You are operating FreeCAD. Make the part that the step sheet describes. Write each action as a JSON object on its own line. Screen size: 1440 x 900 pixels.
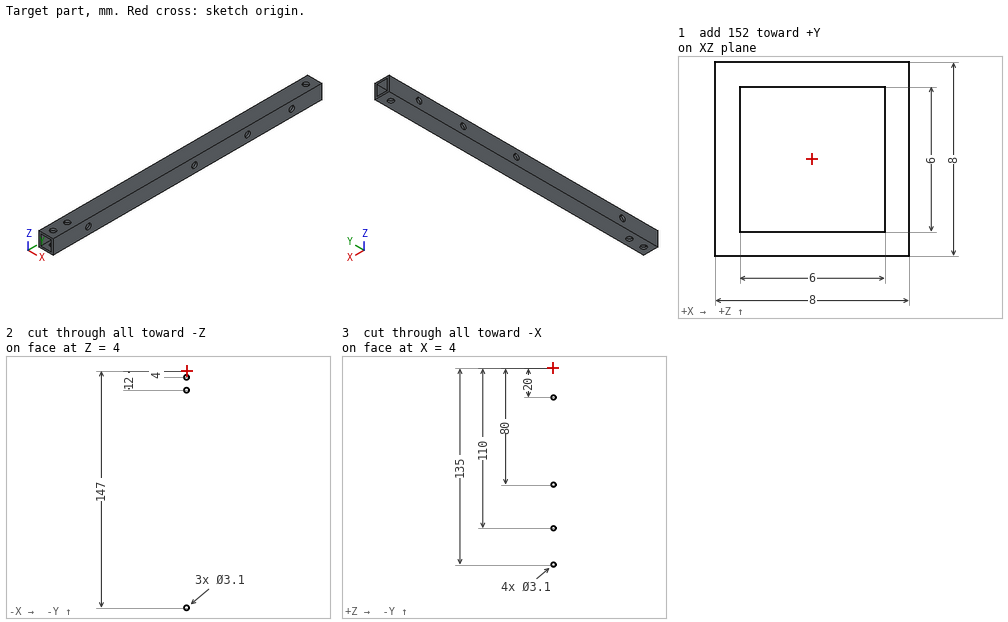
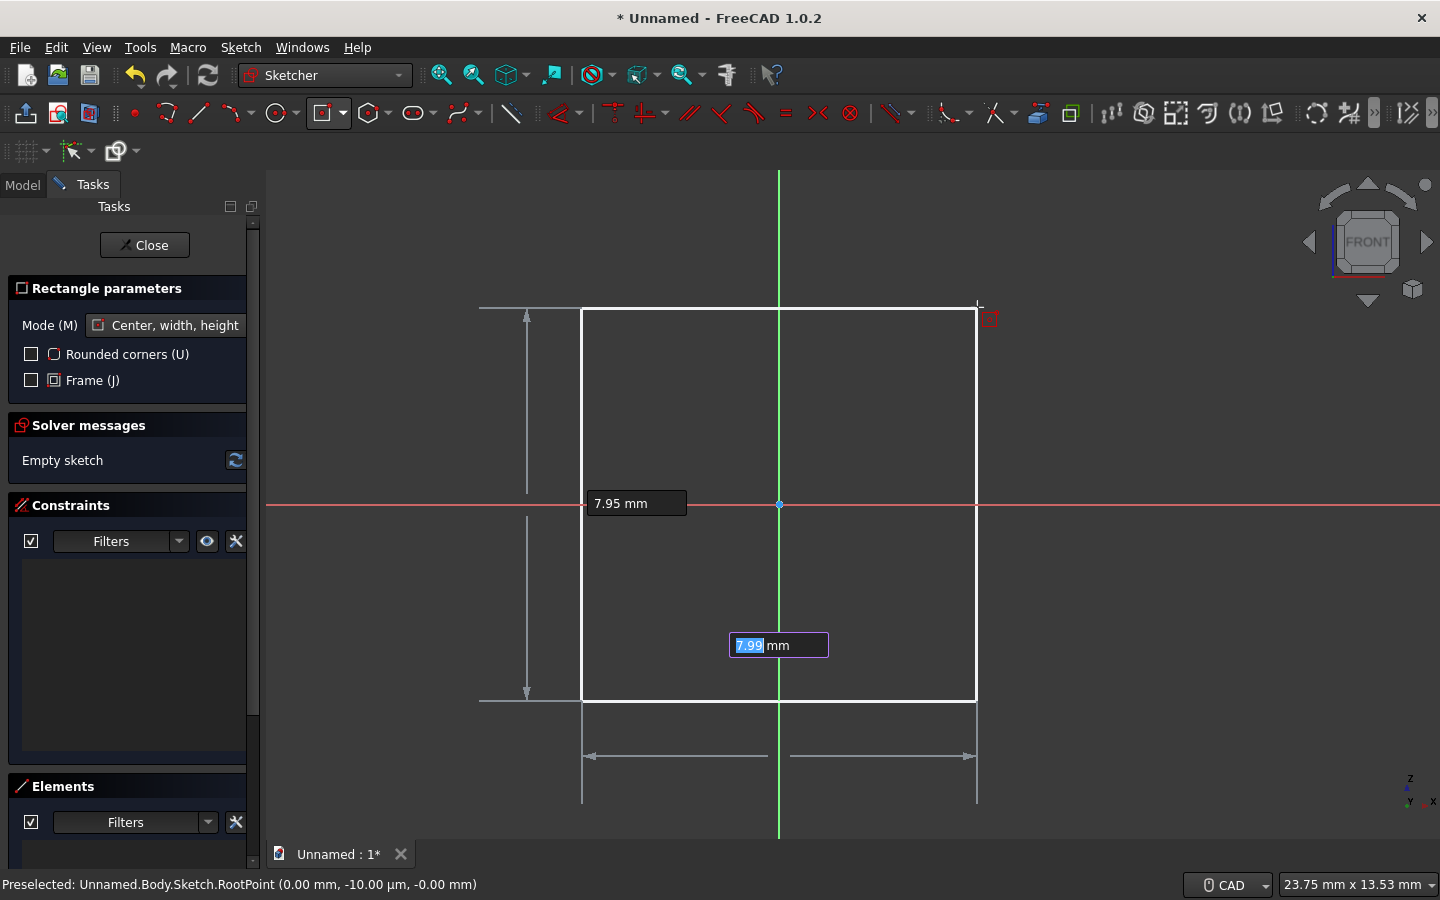
{"action": "type", "text": "8"}
{"action": "key", "text": "Tab"}
{"action": "type", "text": "8"}
{"action": "key", "text": "Return"}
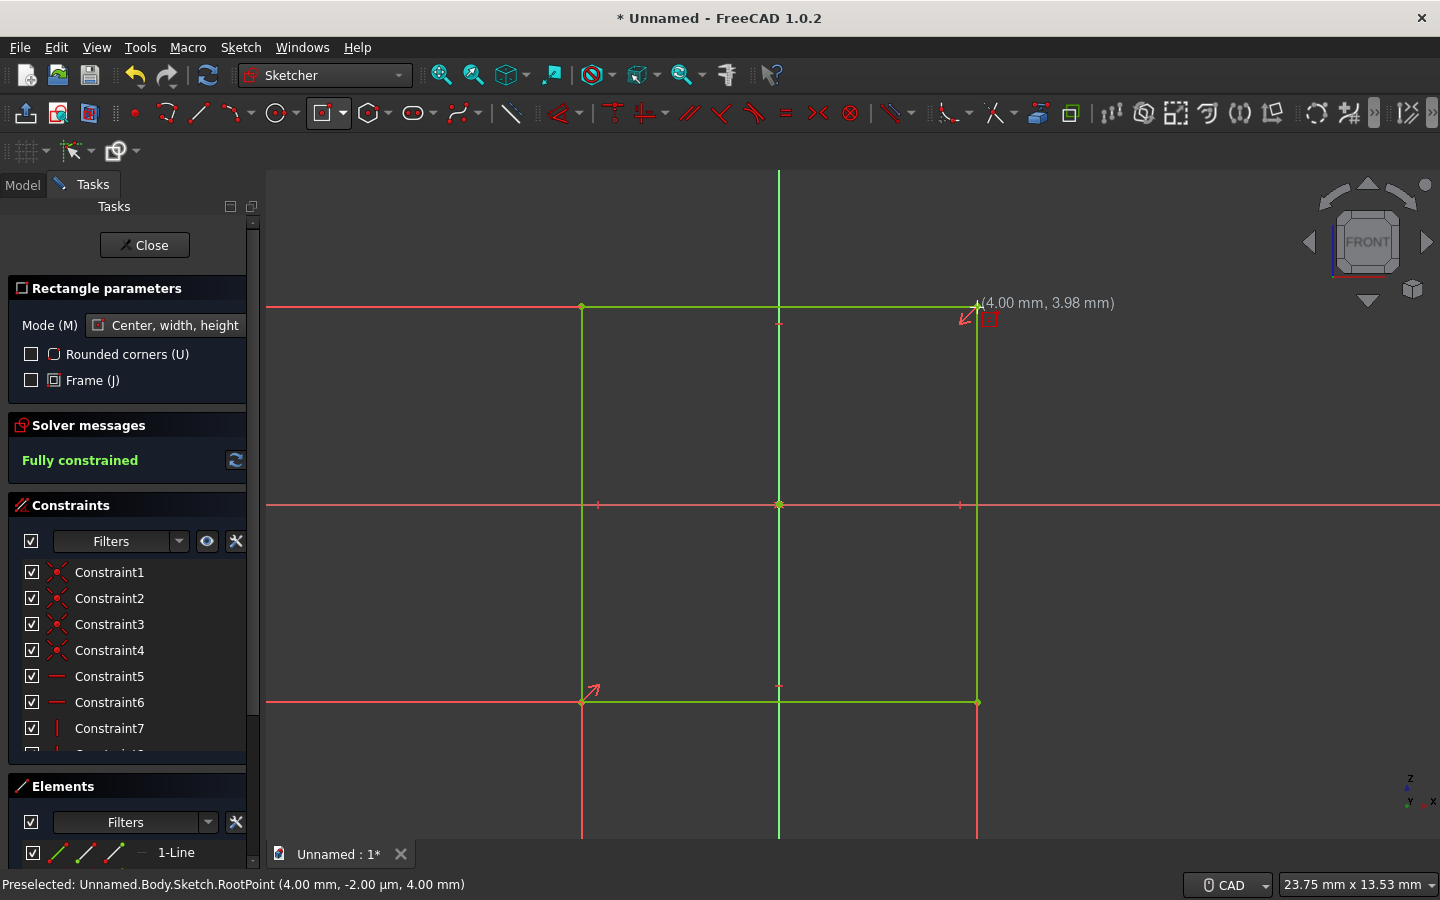
{"action": "left_click", "coordinate": [779, 504]}
{"action": "mouse_move", "coordinate": [928, 356]}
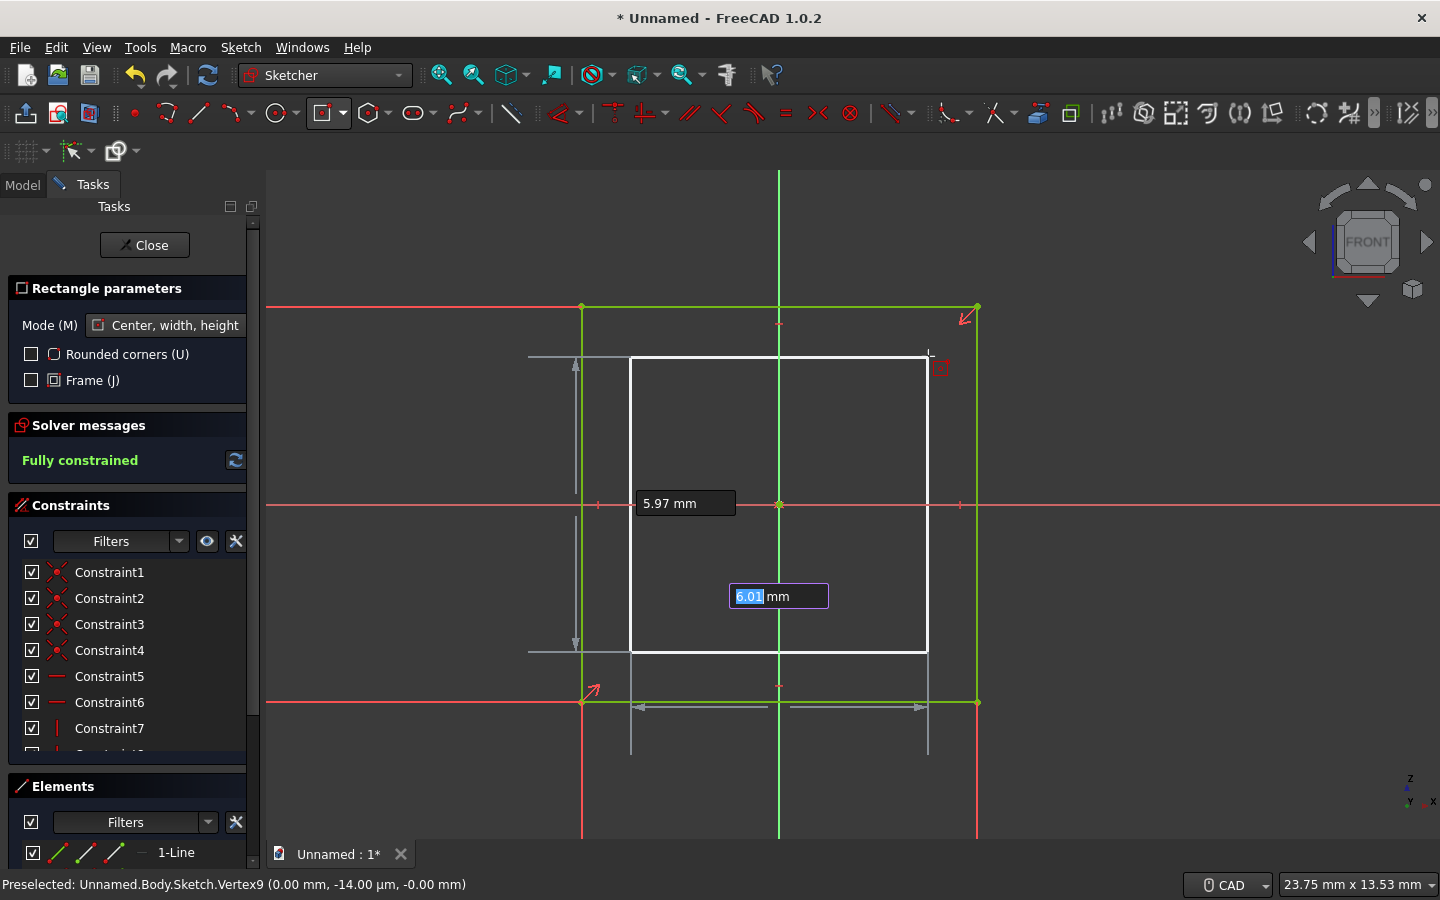
{"action": "type", "text": "6"}
{"action": "key", "text": "Tab"}
{"action": "type", "text": "6"}
{"action": "key", "text": "Return"}
{"action": "key", "text": "Escape"}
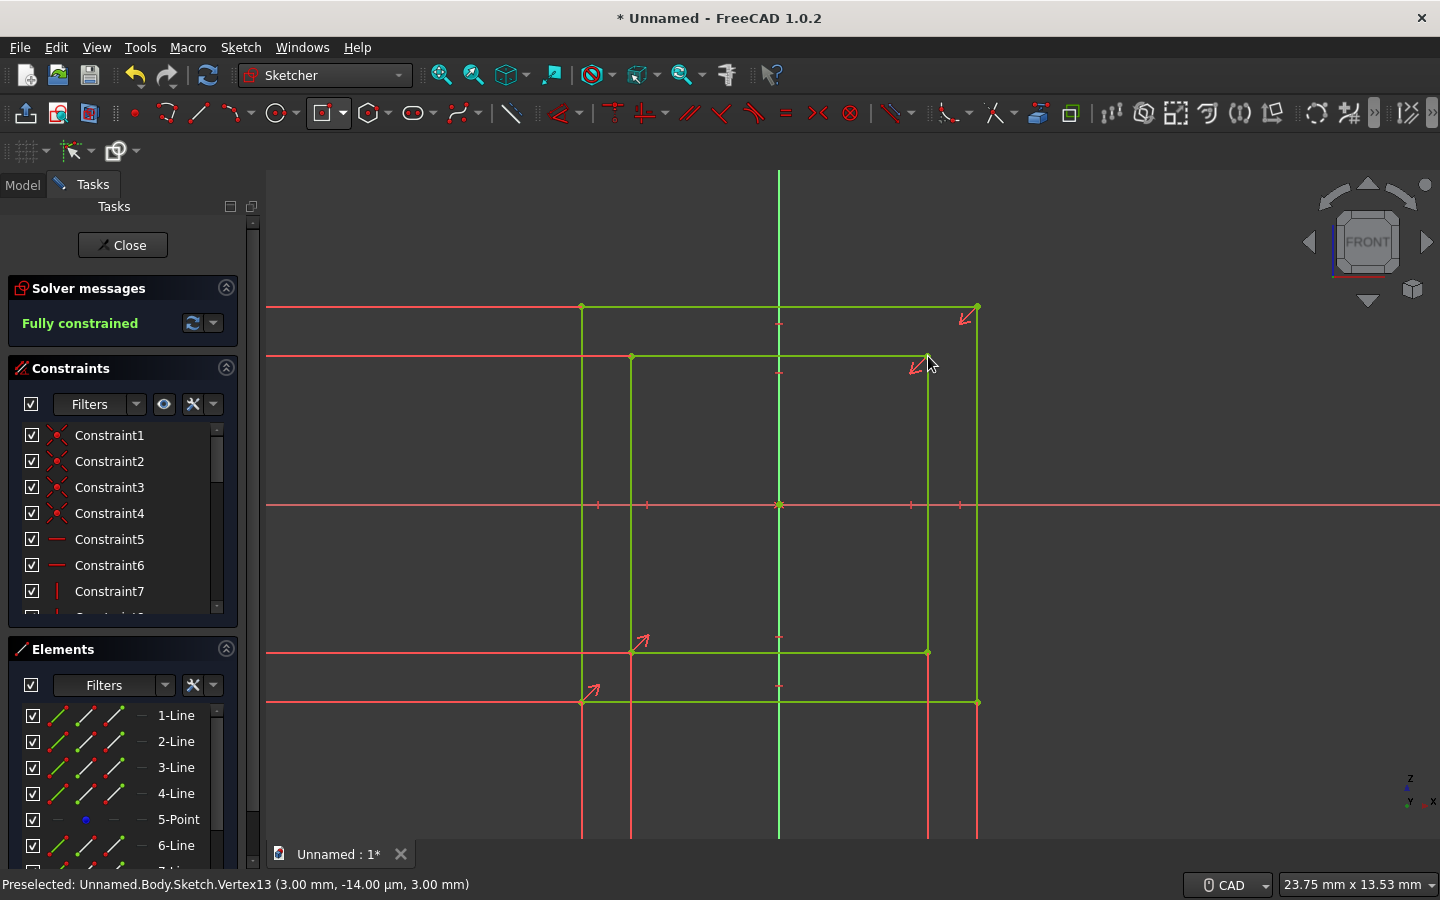
{"action": "left_click", "coordinate": [123, 245]}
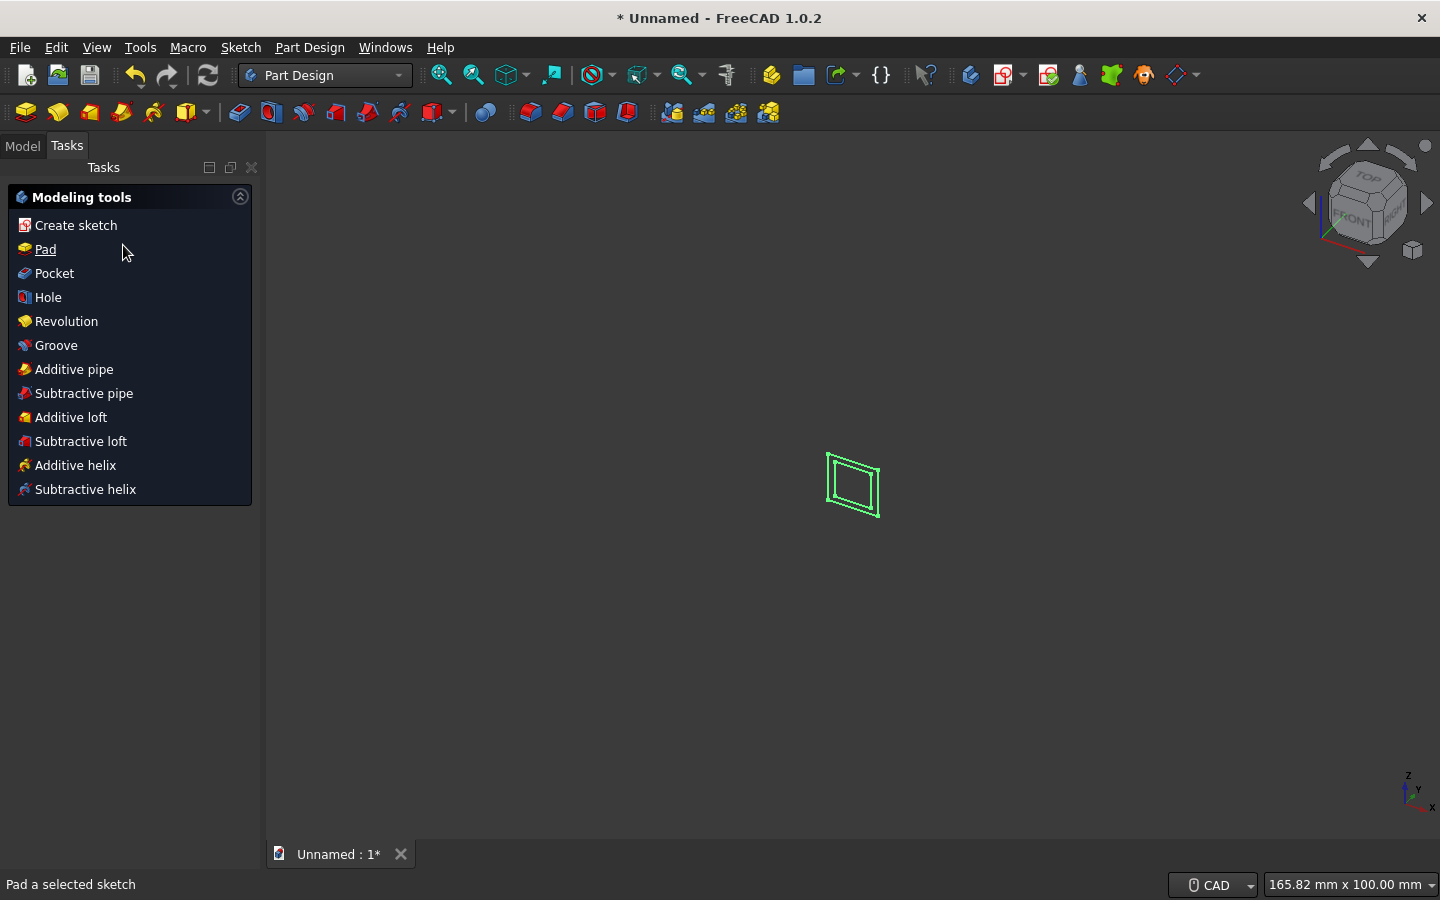
{"action": "left_click", "coordinate": [26, 112]}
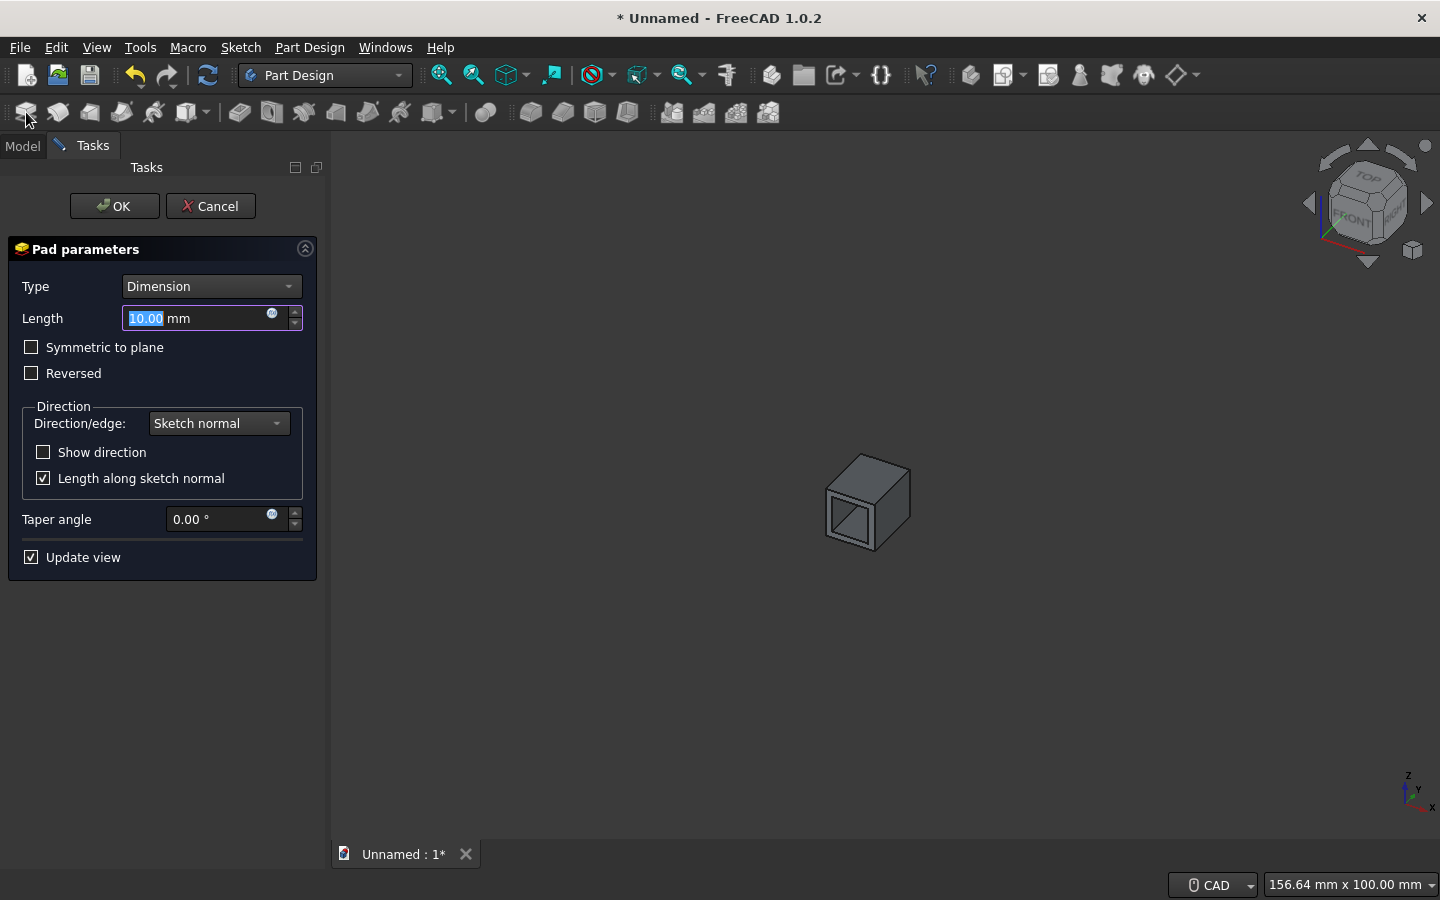
{"action": "type", "text": "152"}
{"action": "key", "text": "Tab"}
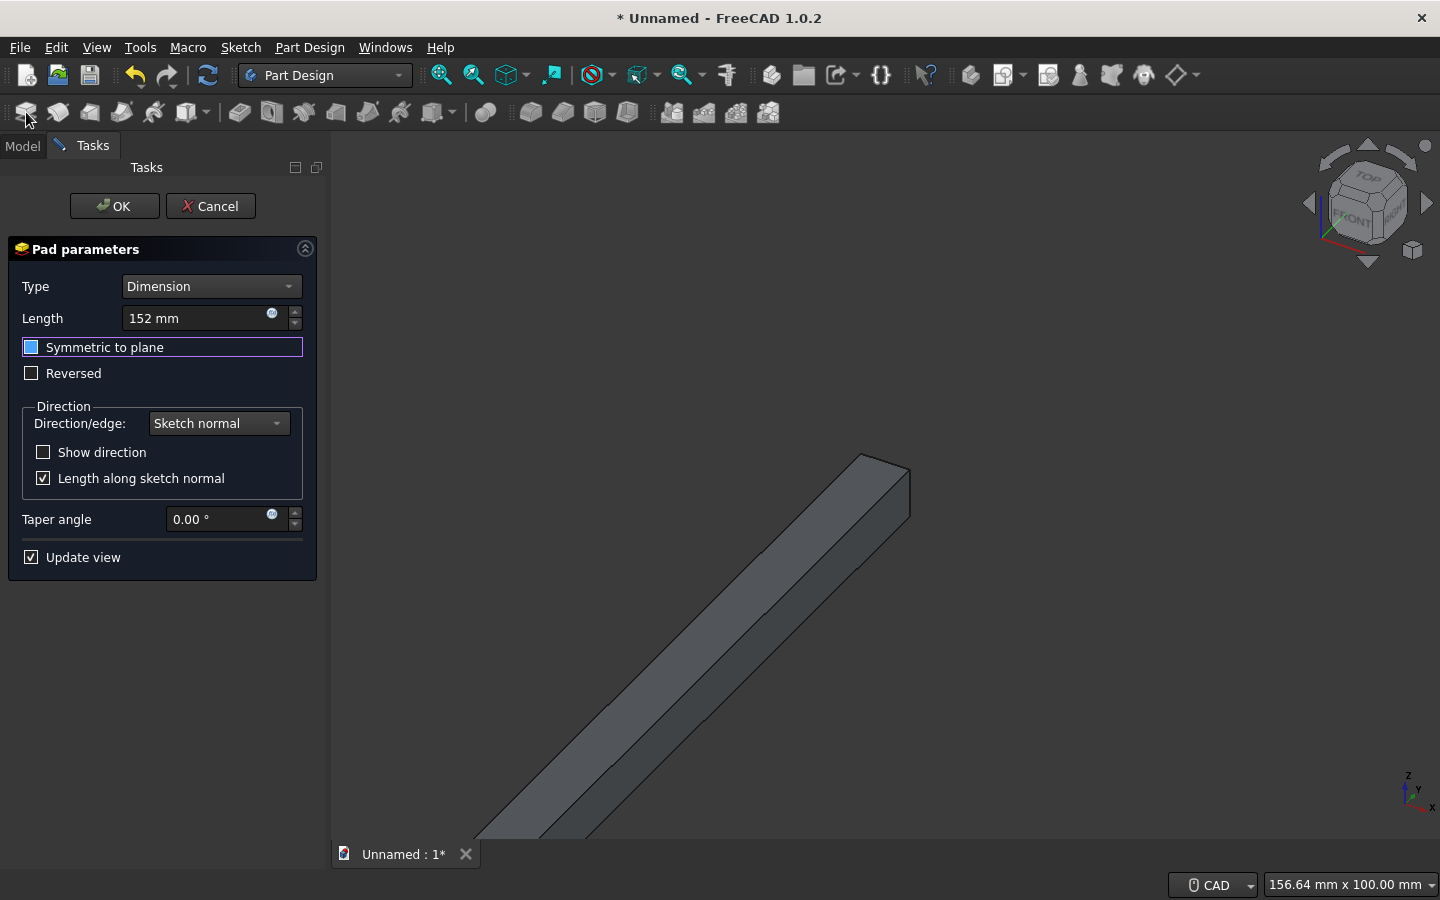
{"action": "left_click", "coordinate": [30, 373]}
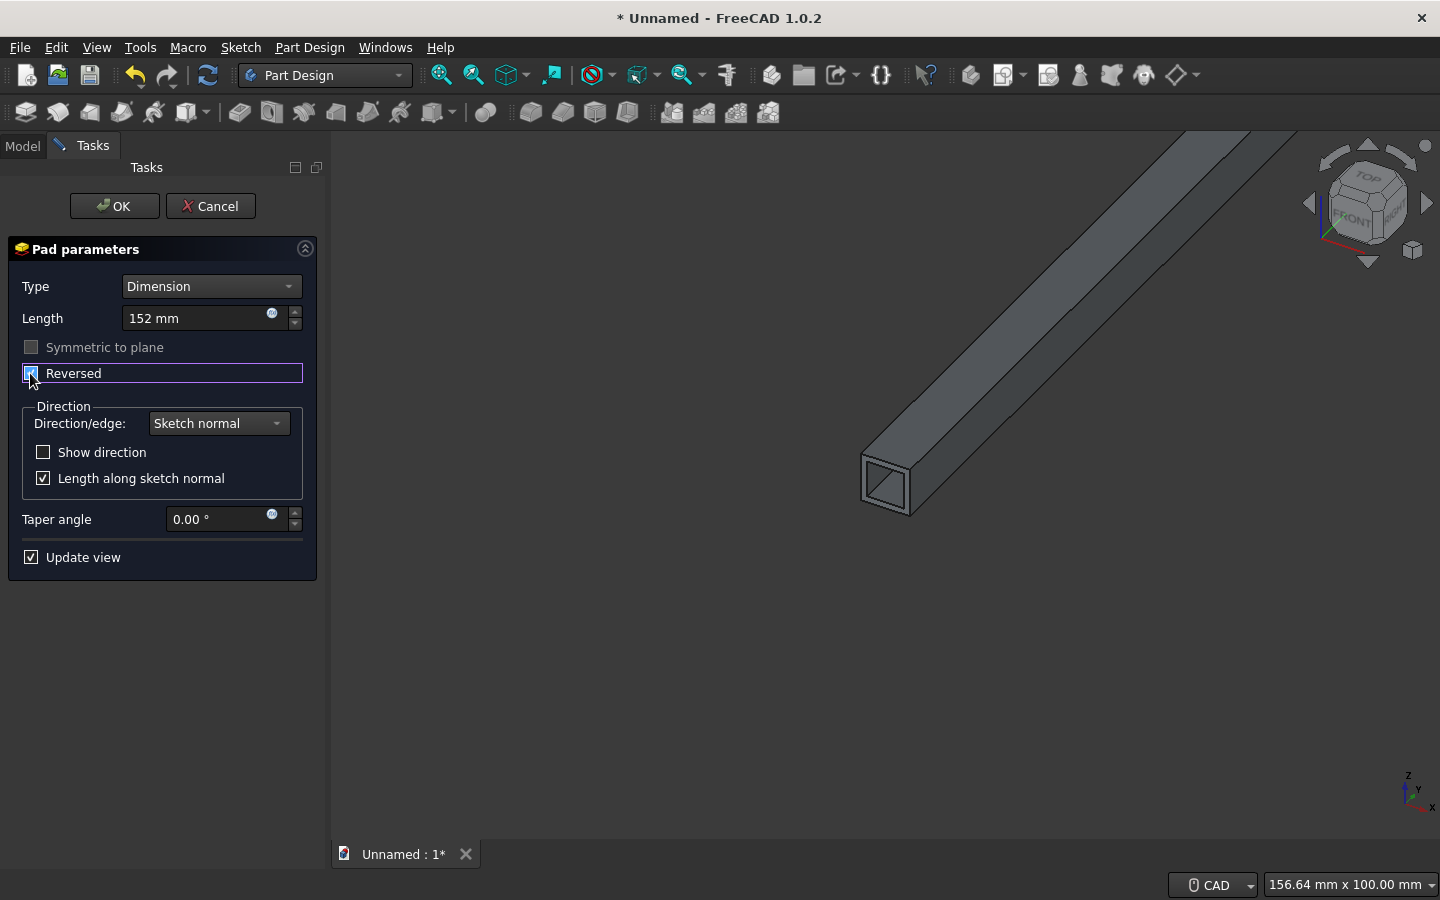
{"action": "left_click", "coordinate": [115, 206]}